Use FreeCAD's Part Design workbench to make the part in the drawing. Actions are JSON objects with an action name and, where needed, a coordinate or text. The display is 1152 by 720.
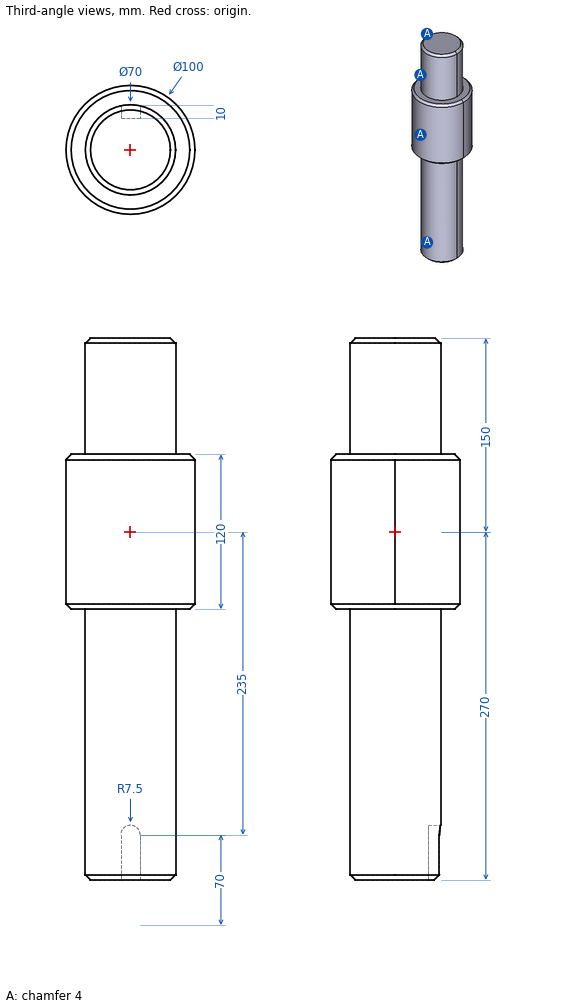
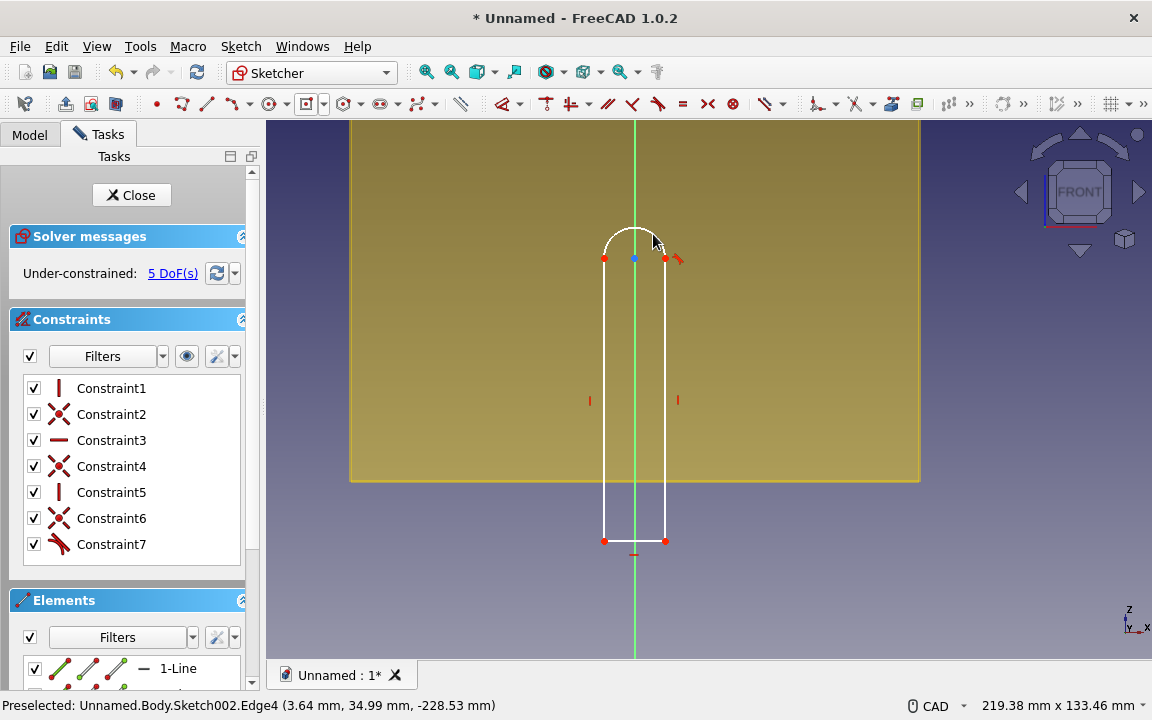
{"action": "left_click", "coordinate": [604, 456]}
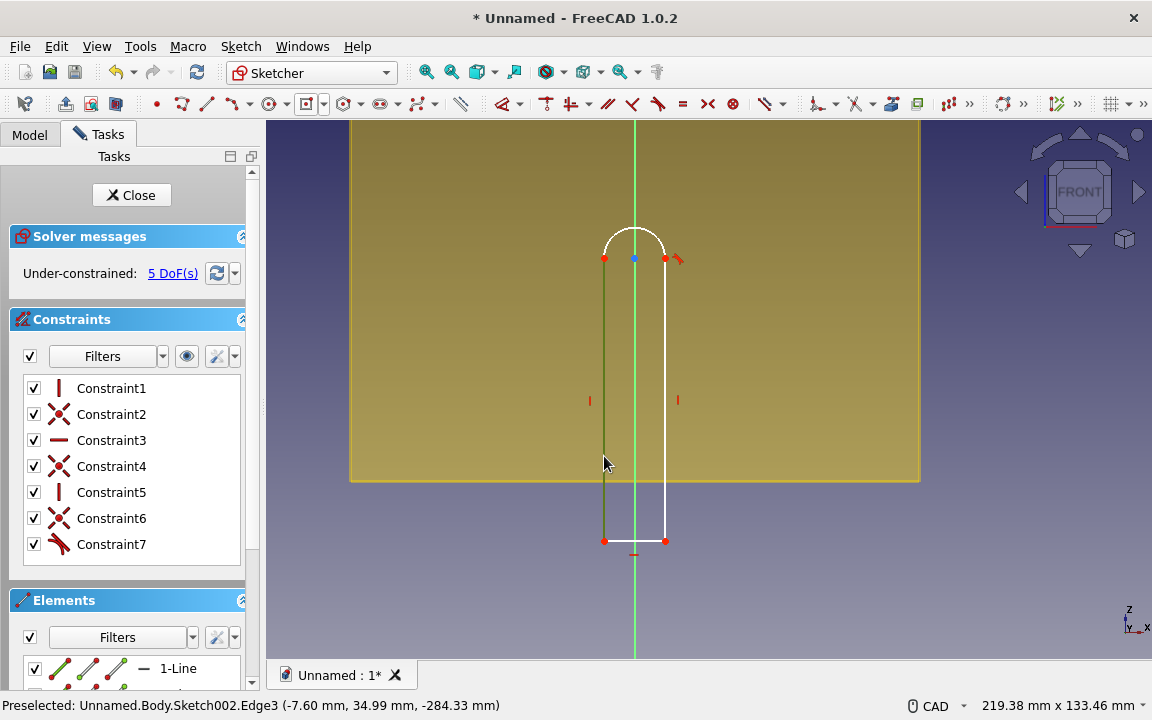
{"action": "left_click", "coordinate": [652, 233]}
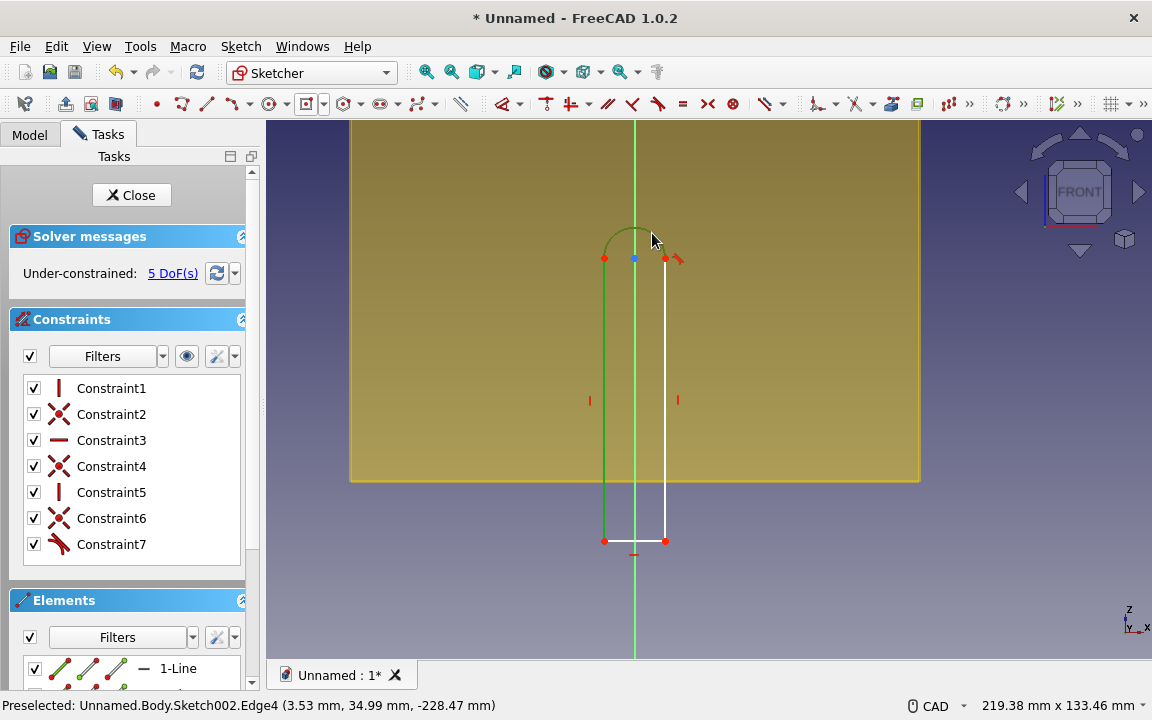
{"action": "key", "text": "t"}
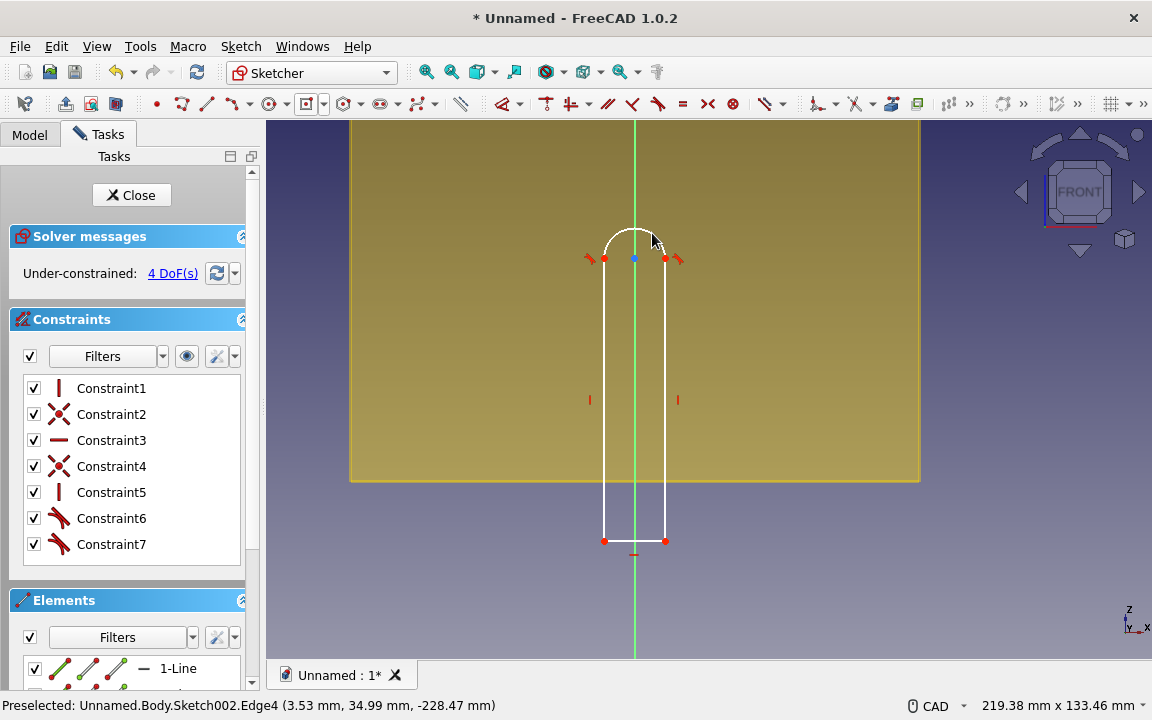
{"action": "left_click", "coordinate": [634, 259]}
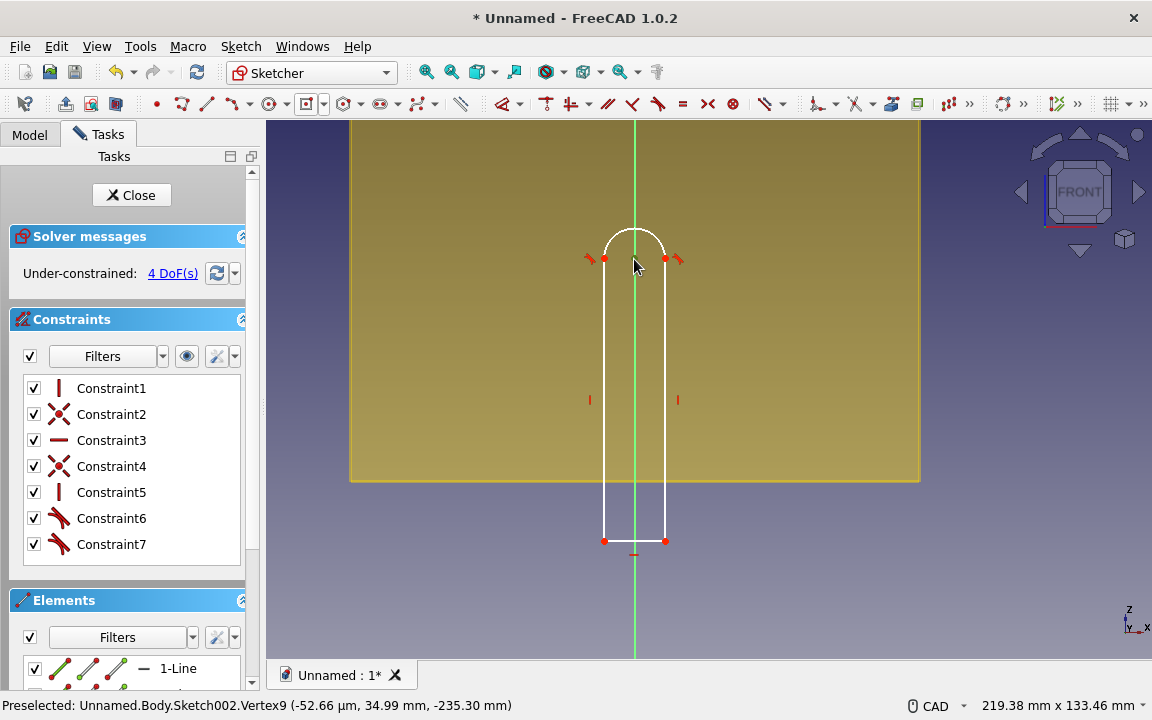
{"action": "left_click", "coordinate": [635, 596]}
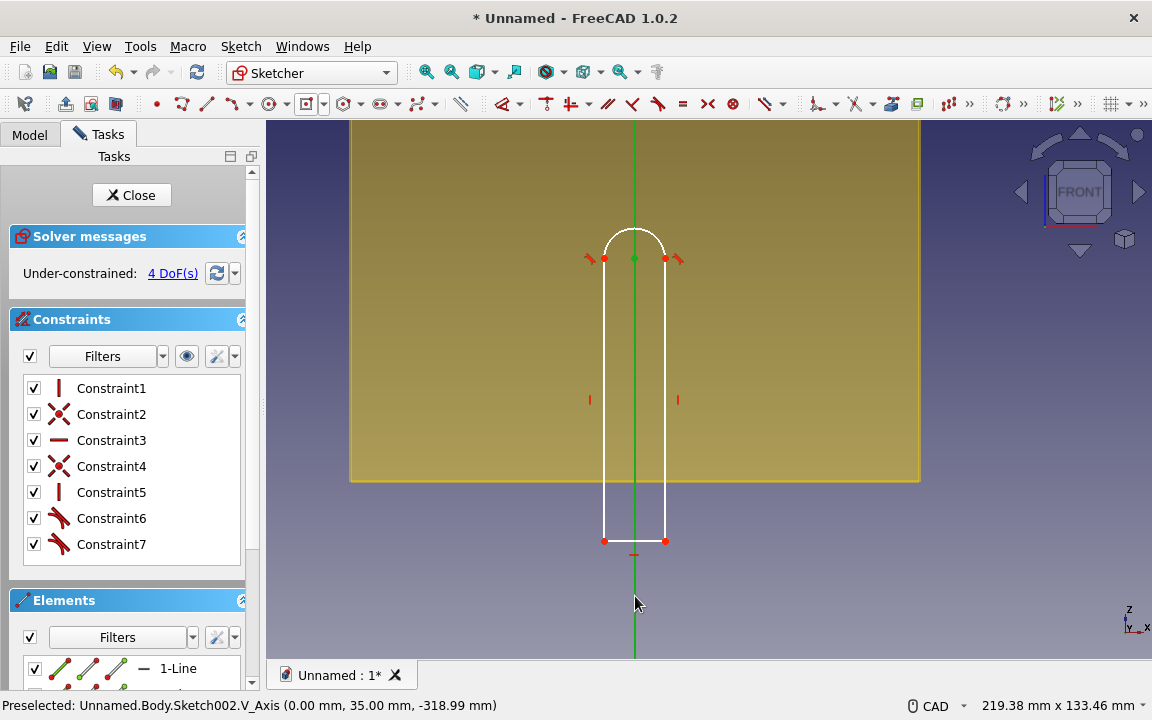
{"action": "key", "text": "c"}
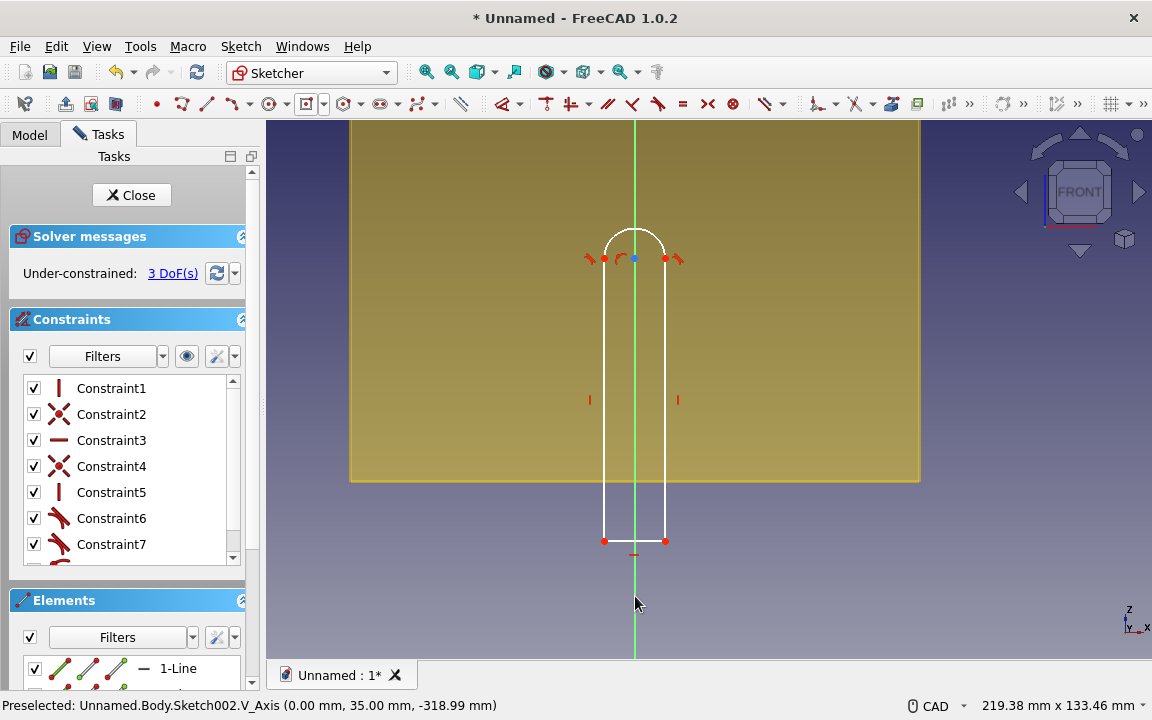
{"action": "key", "text": "d"}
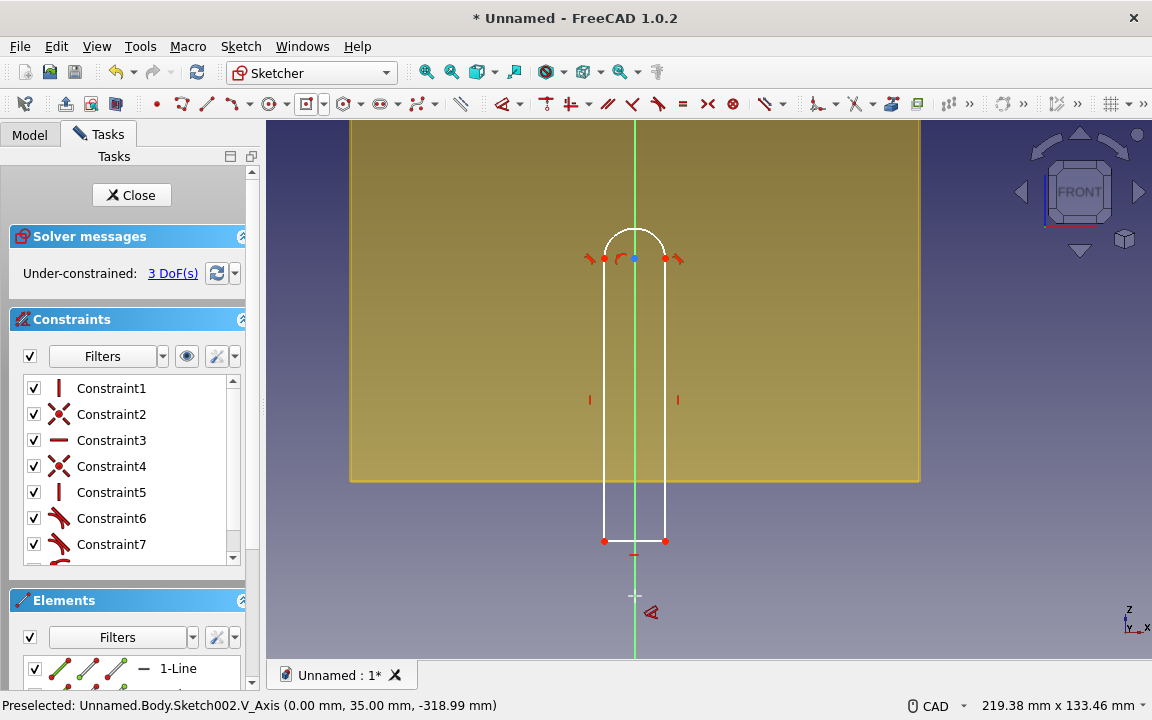
{"action": "scroll", "coordinate": [653, 234], "scroll_direction": "up", "scroll_amount": 2}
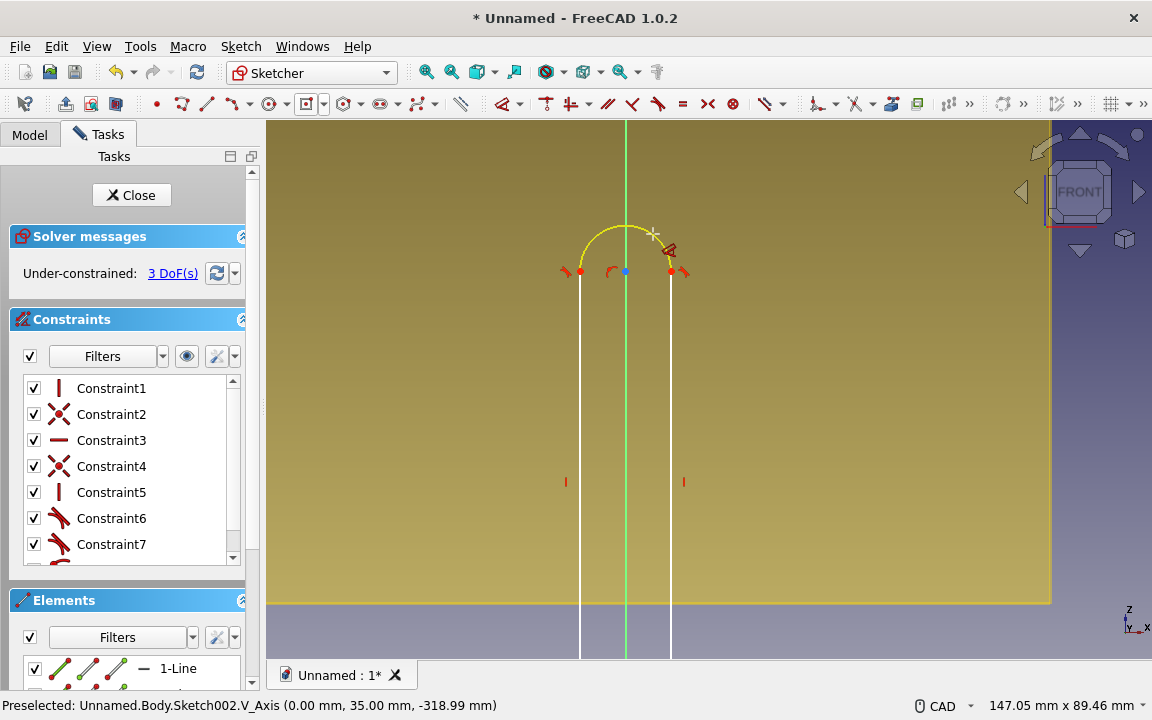
{"action": "left_click", "coordinate": [652, 234]}
{"action": "left_click", "coordinate": [671, 208]}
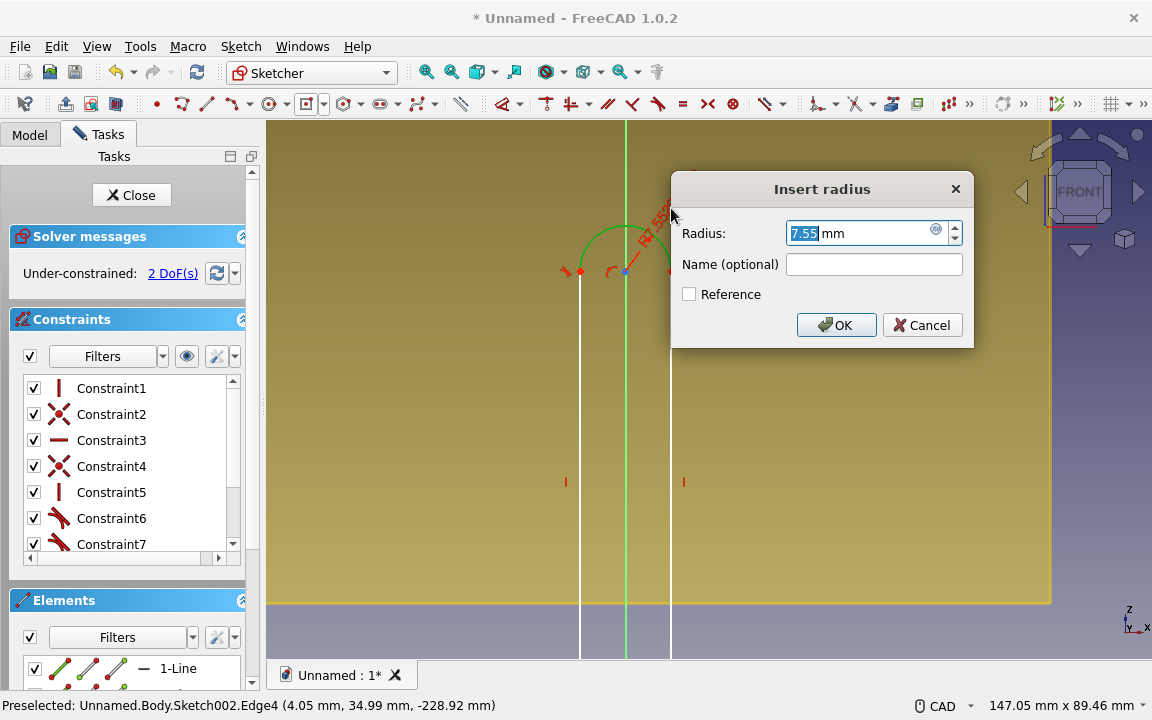
{"action": "type", "text": "7.5"}
{"action": "key", "text": "Return"}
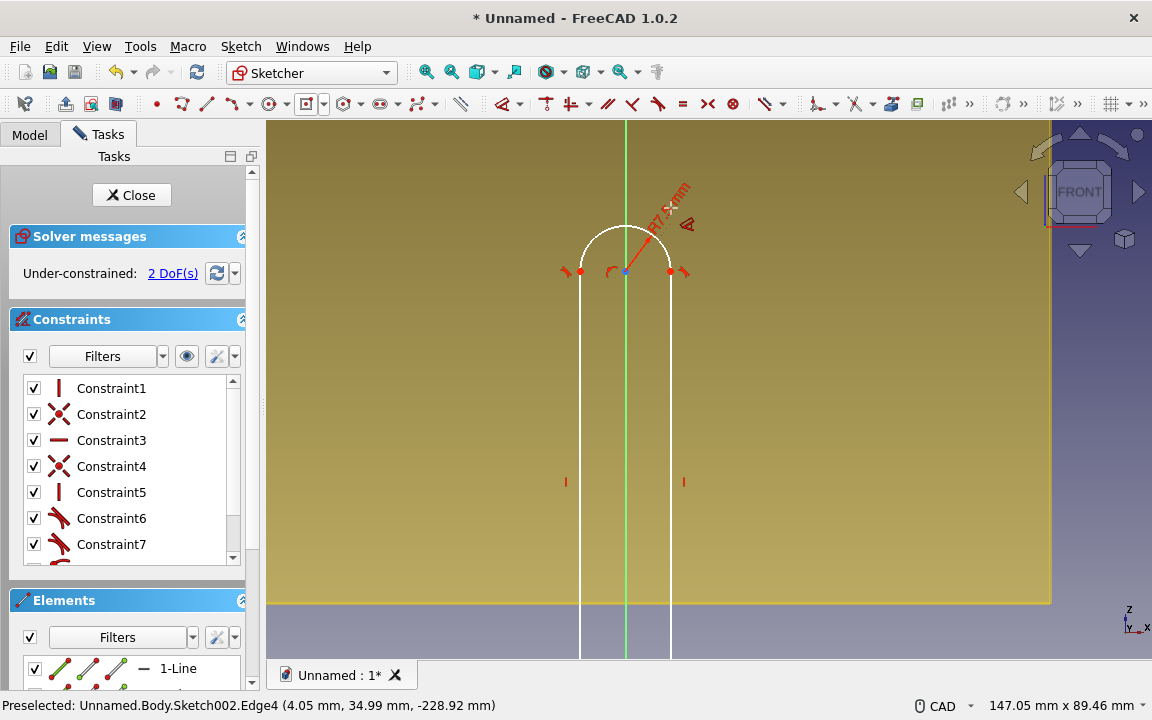
{"action": "left_click", "coordinate": [671, 397]}
{"action": "left_click", "coordinate": [705, 451]}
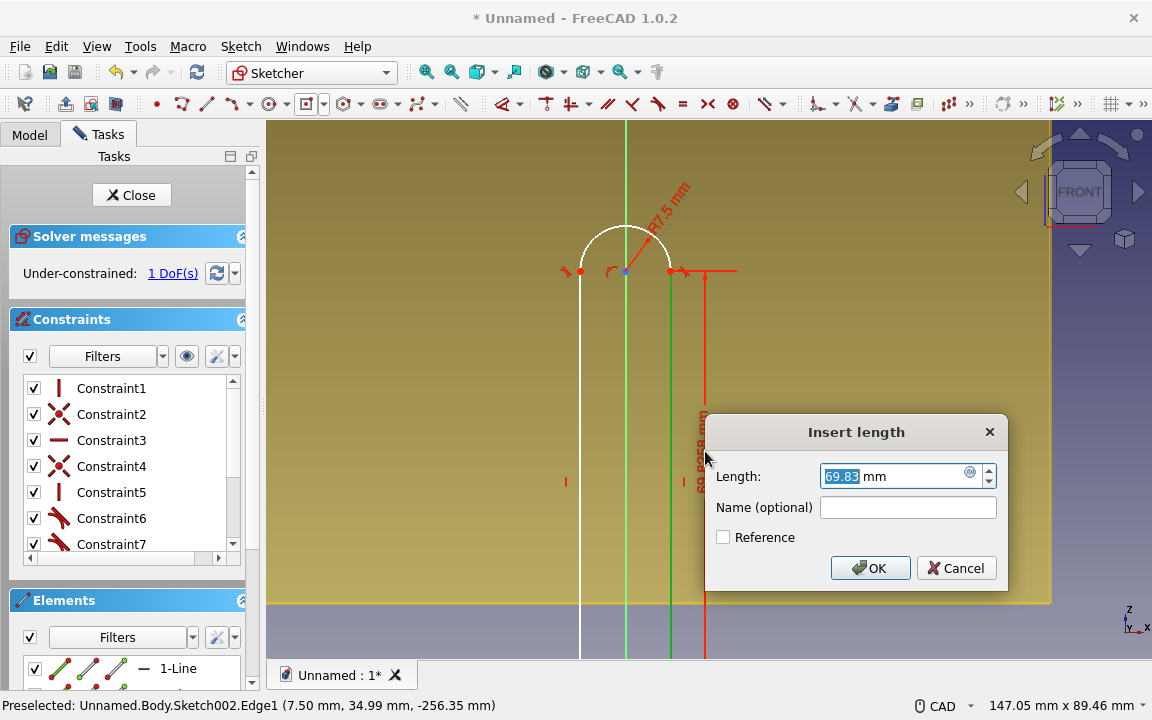
{"action": "type", "text": "70"}
{"action": "key", "text": "Return"}